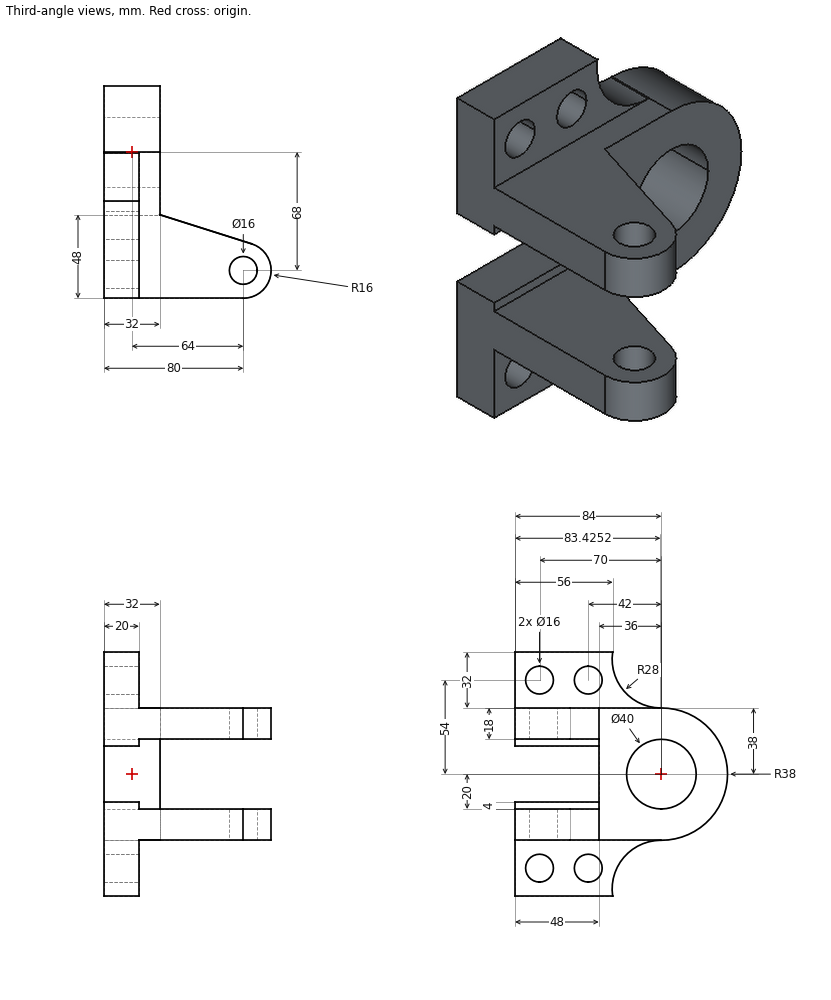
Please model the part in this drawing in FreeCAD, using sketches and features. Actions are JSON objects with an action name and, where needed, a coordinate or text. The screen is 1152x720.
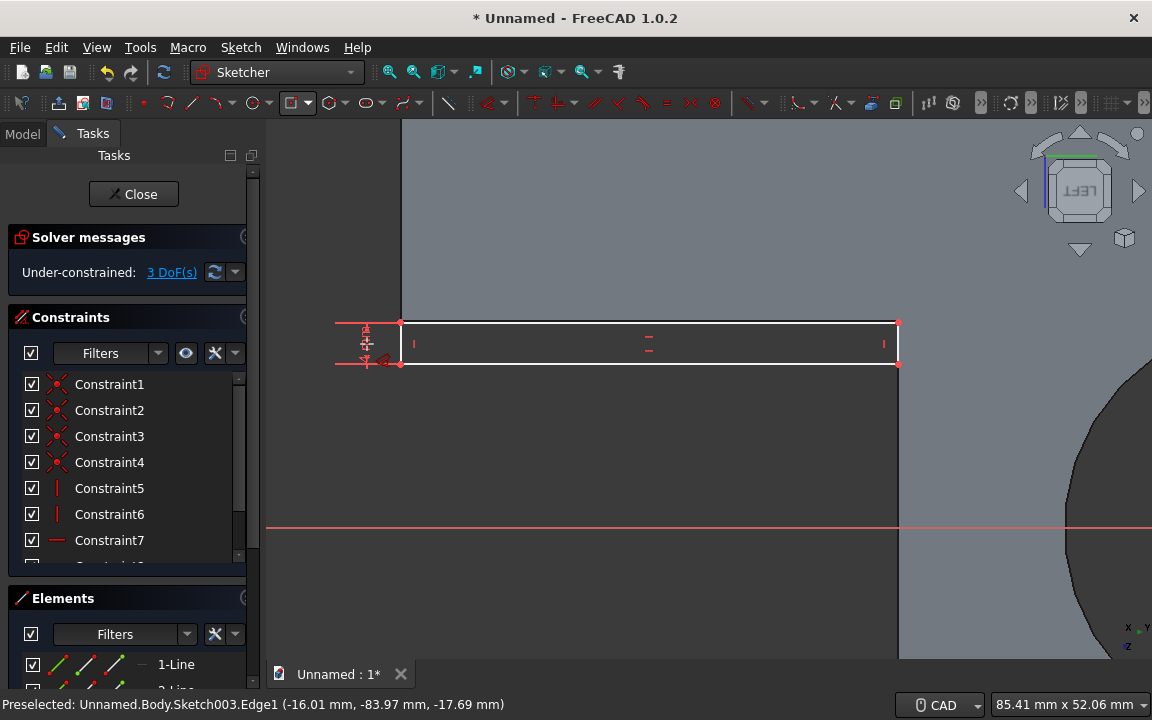
{"action": "left_click", "coordinate": [550, 364]}
{"action": "left_click", "coordinate": [650, 398]}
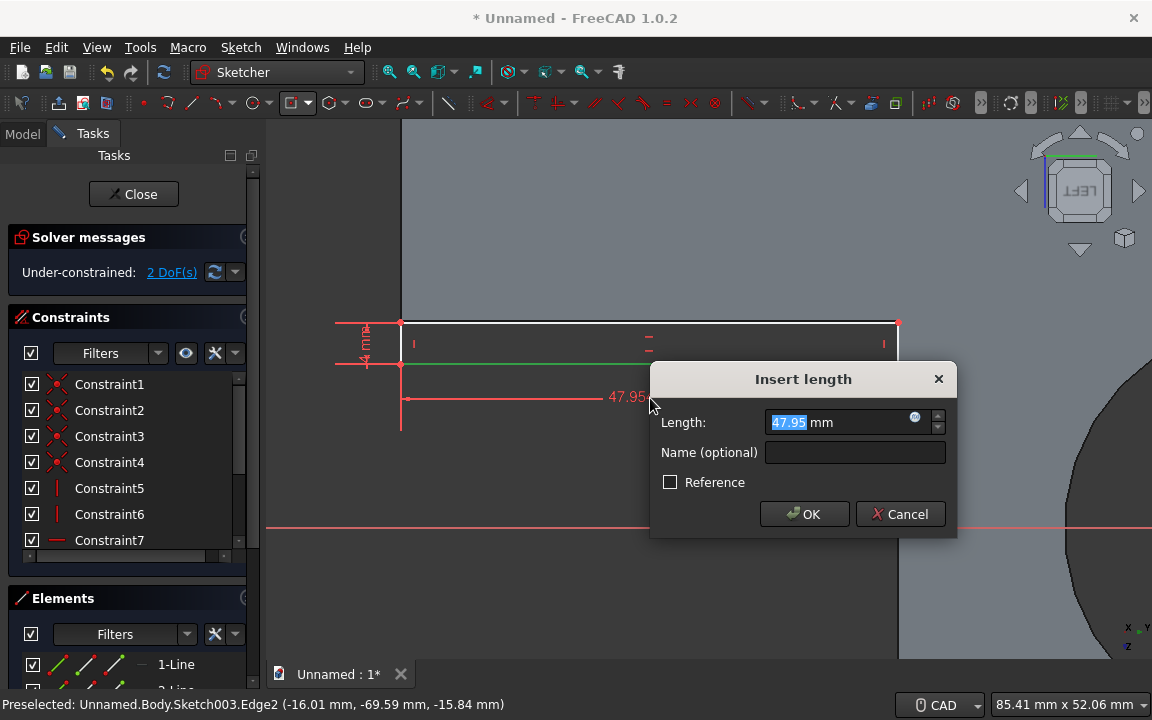
{"action": "type", "text": "48"}
{"action": "key", "text": "Return"}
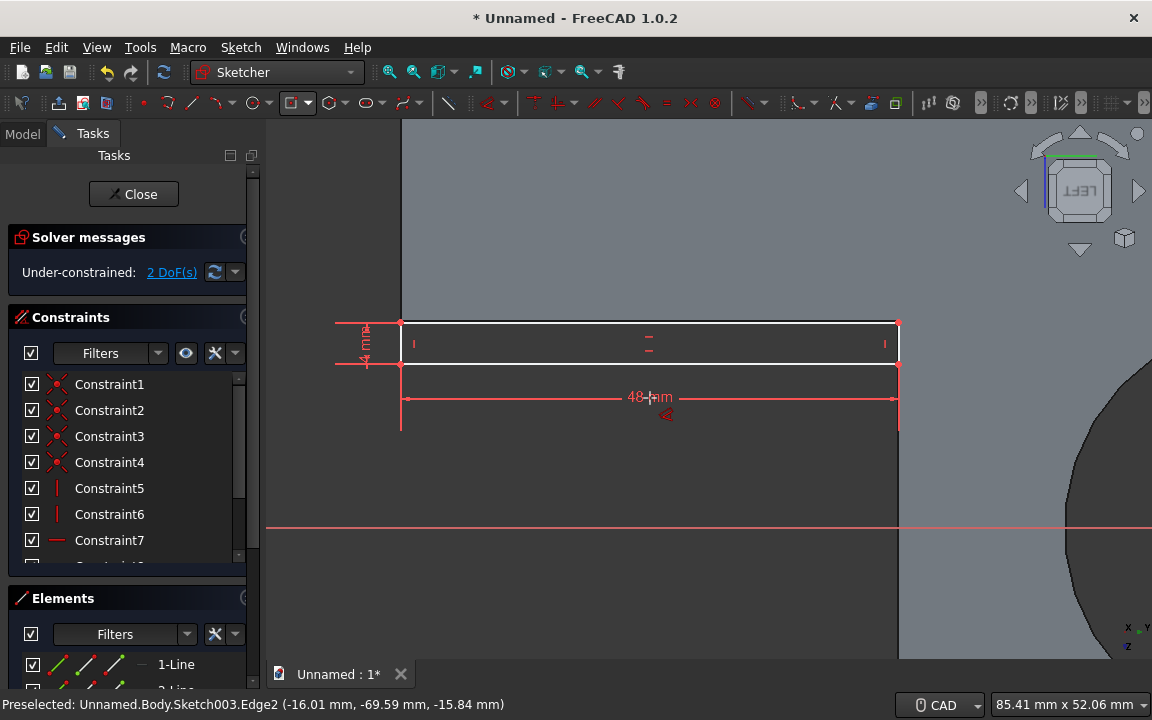
{"action": "left_click", "coordinate": [401, 323]}
{"action": "left_click", "coordinate": [694, 562]}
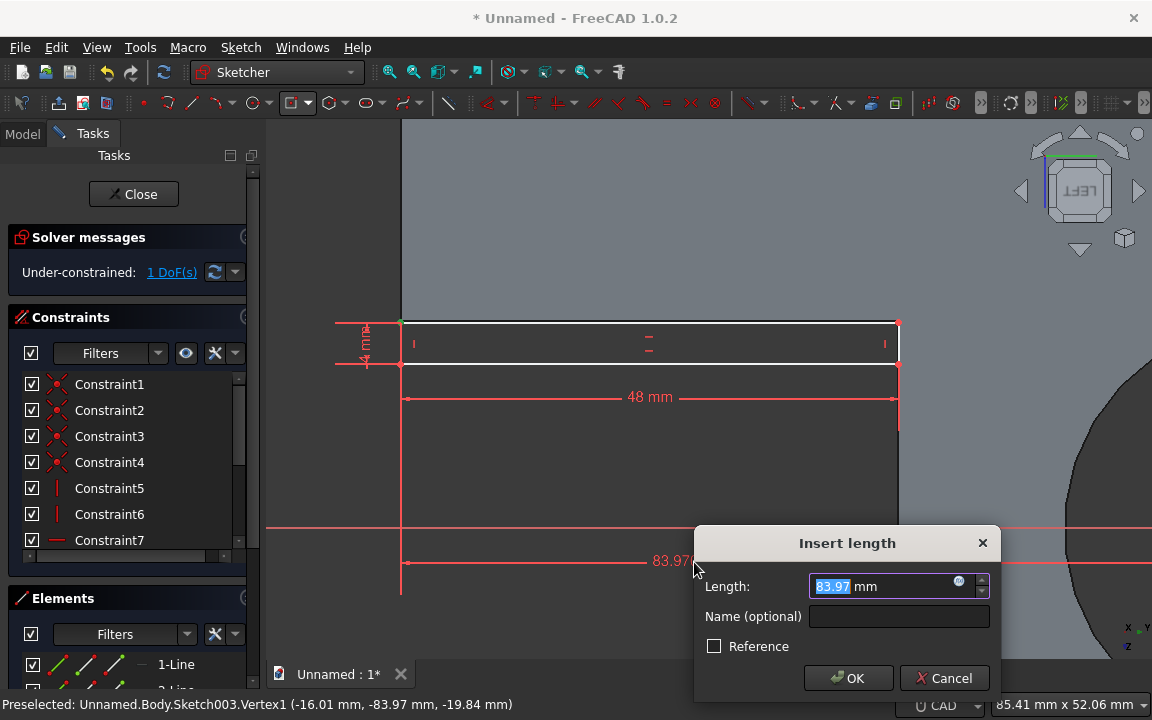
{"action": "type", "text": "84"}
{"action": "key", "text": "Return"}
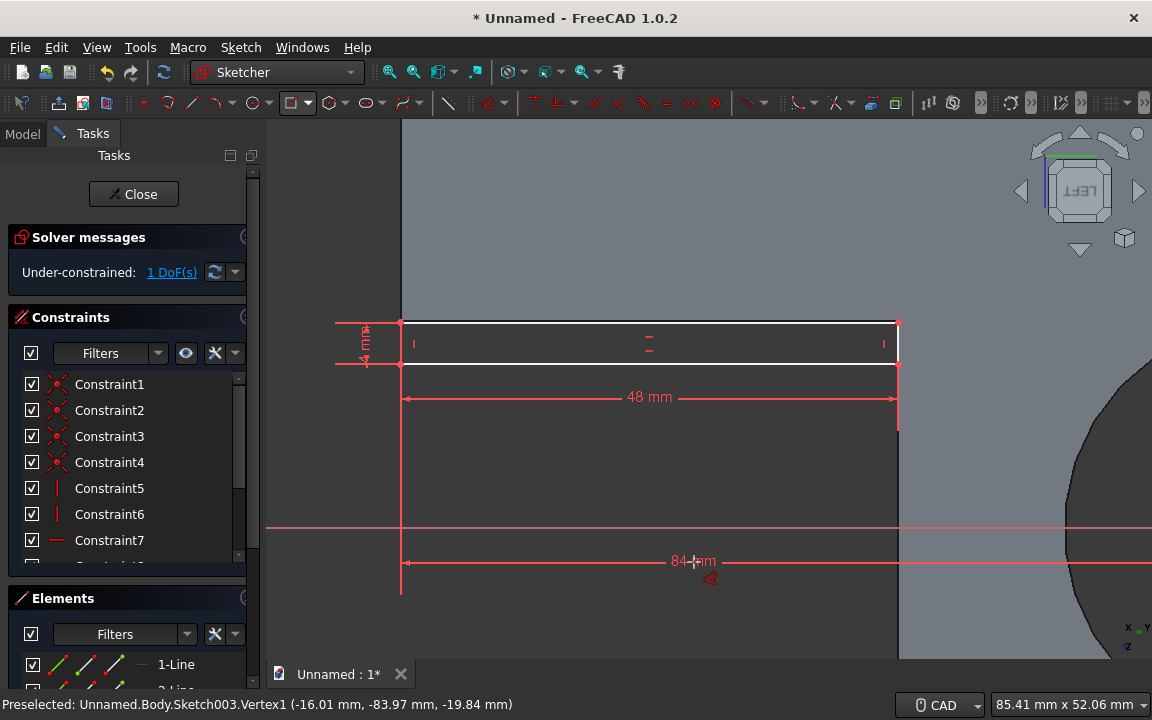
{"action": "left_click", "coordinate": [401, 323]}
{"action": "left_click", "coordinate": [367, 426]}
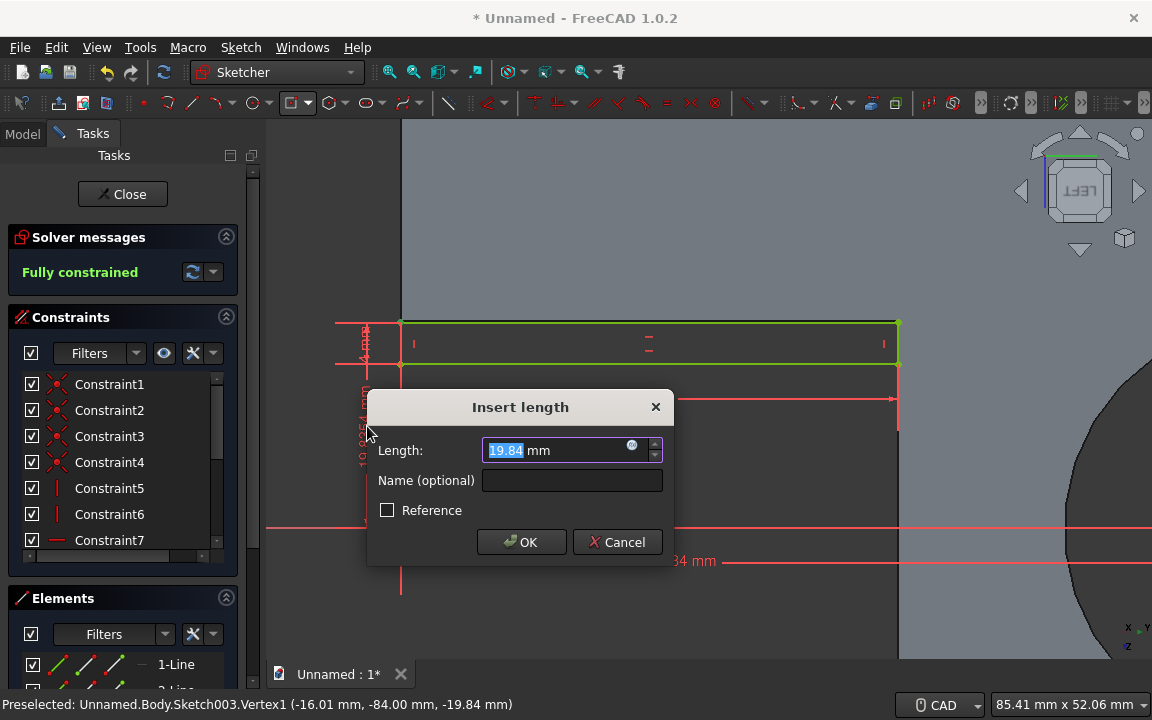
{"action": "type", "text": "20"}
{"action": "key", "text": "Return"}
{"action": "key", "text": "Escape"}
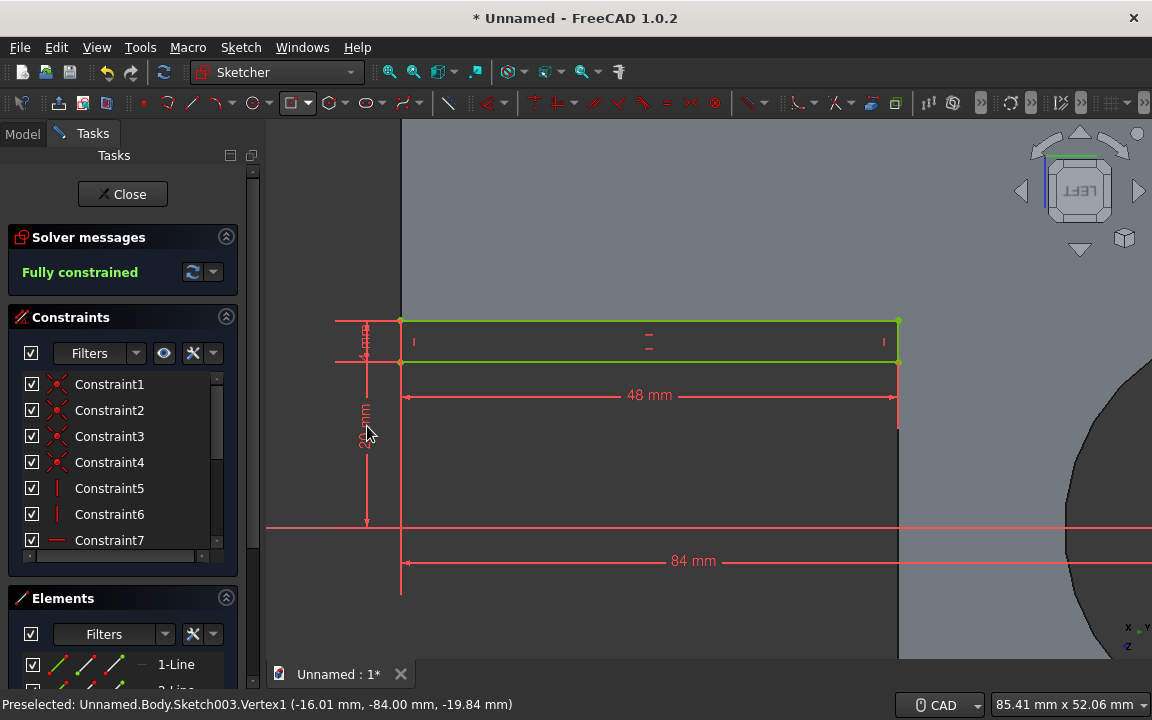
{"action": "left_click", "coordinate": [123, 194]}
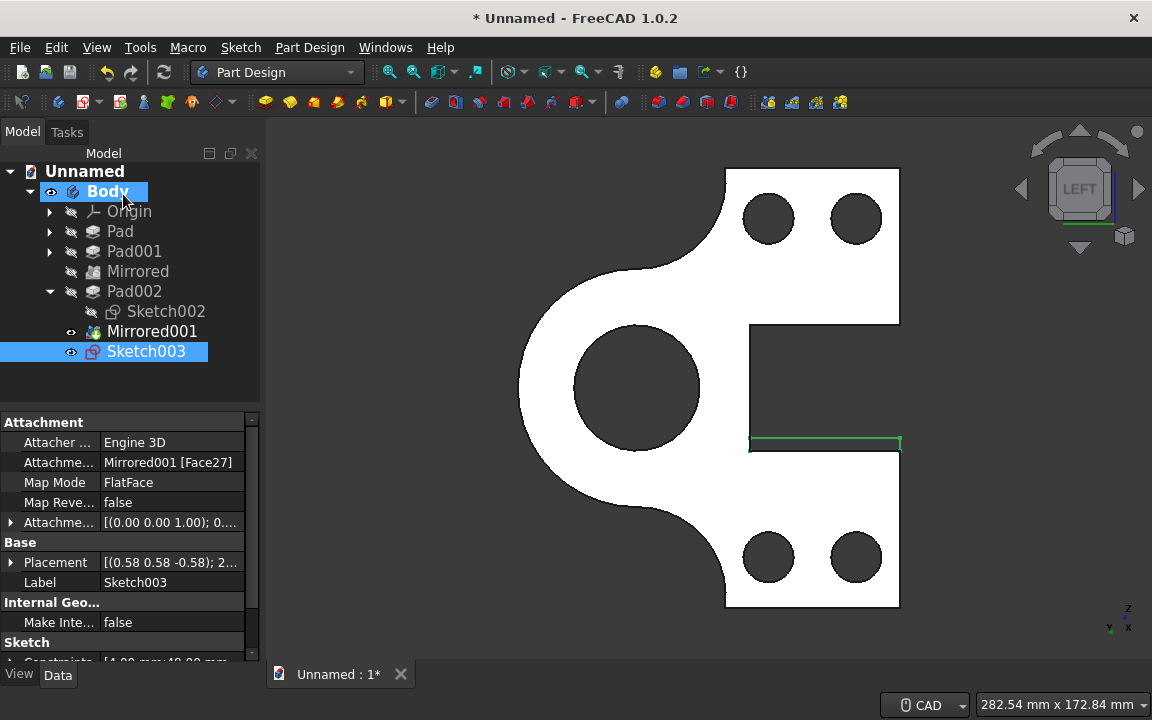
{"action": "left_click", "coordinate": [266, 102]}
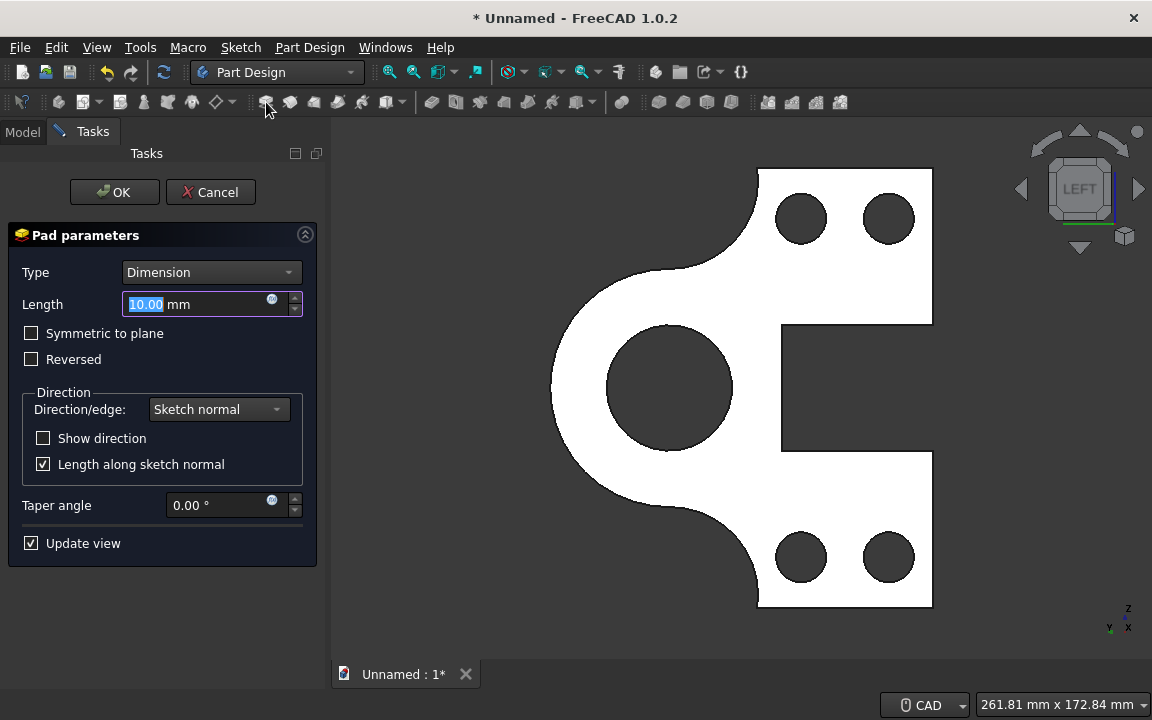
{"action": "type", "text": "20"}
{"action": "key", "text": "Tab"}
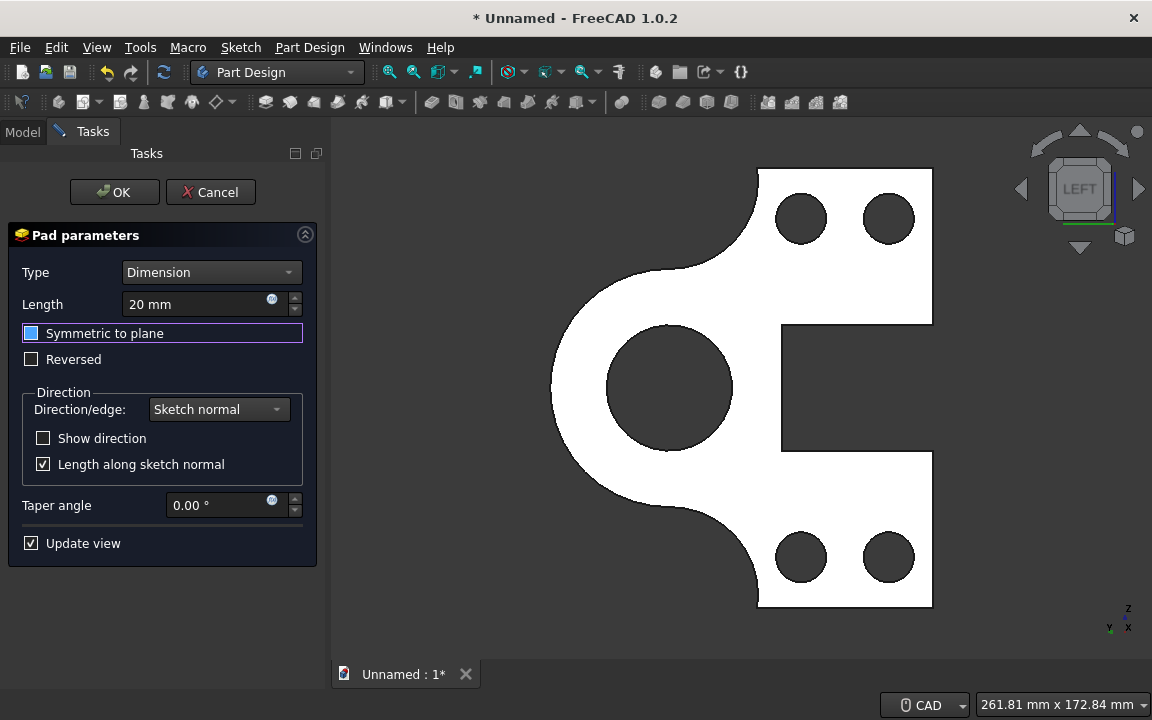
{"action": "left_click", "coordinate": [30, 359]}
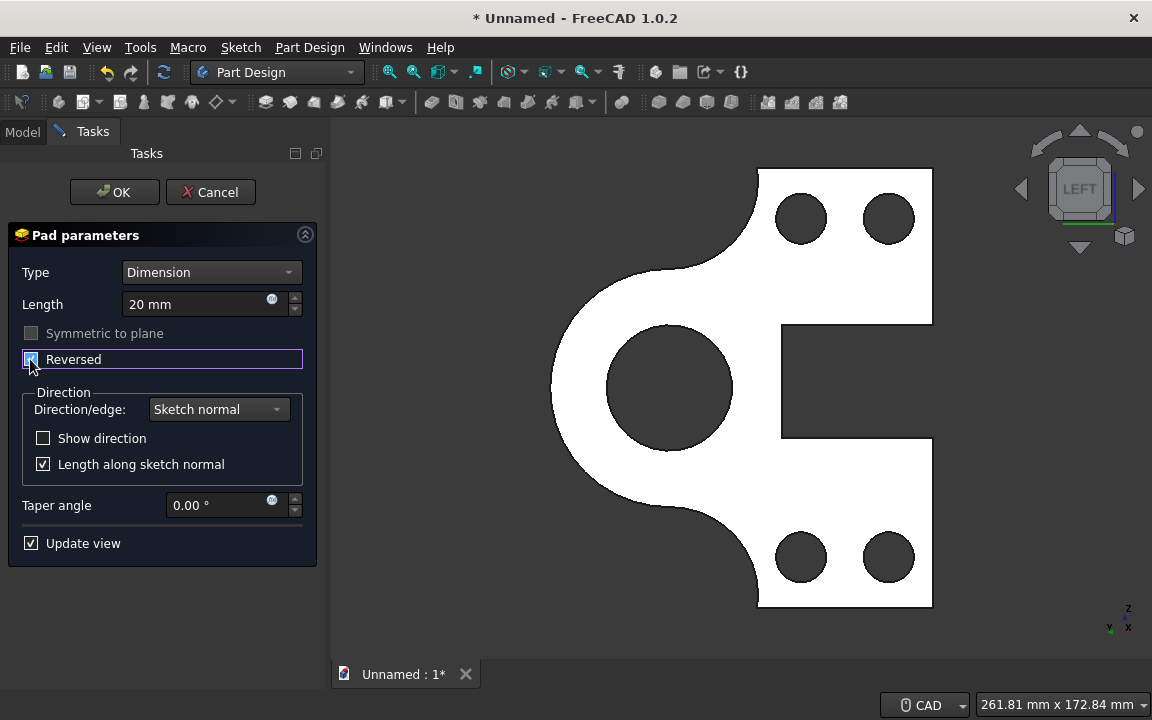
{"action": "left_click", "coordinate": [115, 192]}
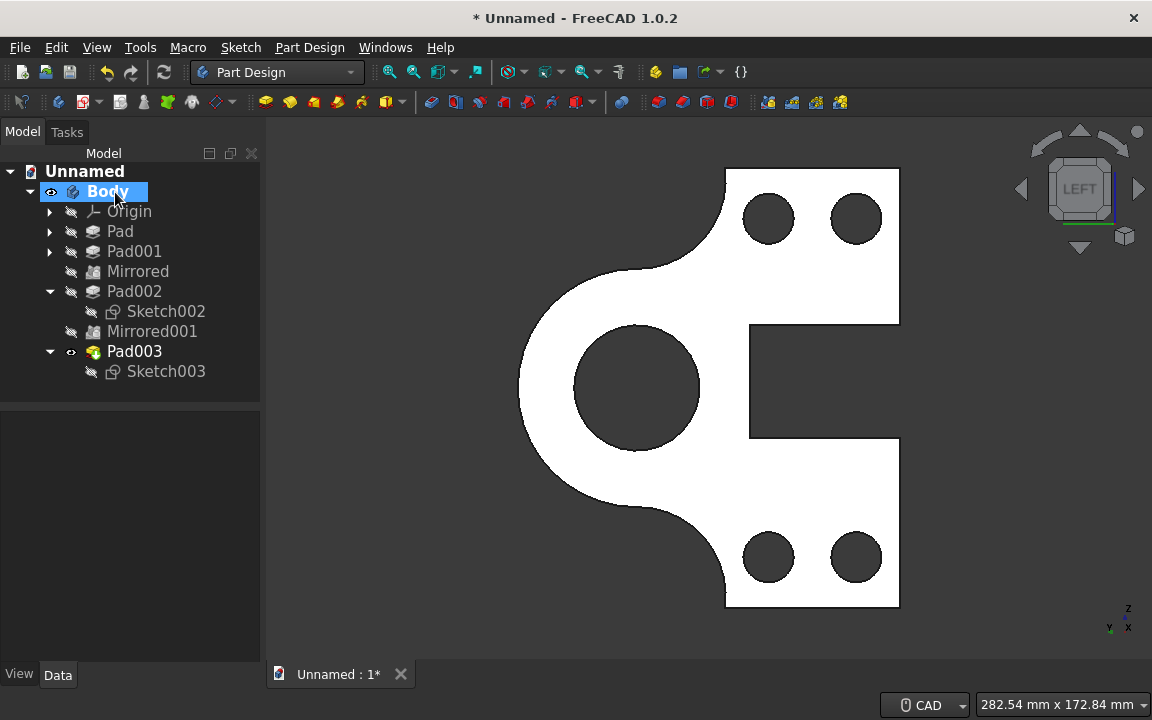
{"action": "left_click", "coordinate": [116, 352]}